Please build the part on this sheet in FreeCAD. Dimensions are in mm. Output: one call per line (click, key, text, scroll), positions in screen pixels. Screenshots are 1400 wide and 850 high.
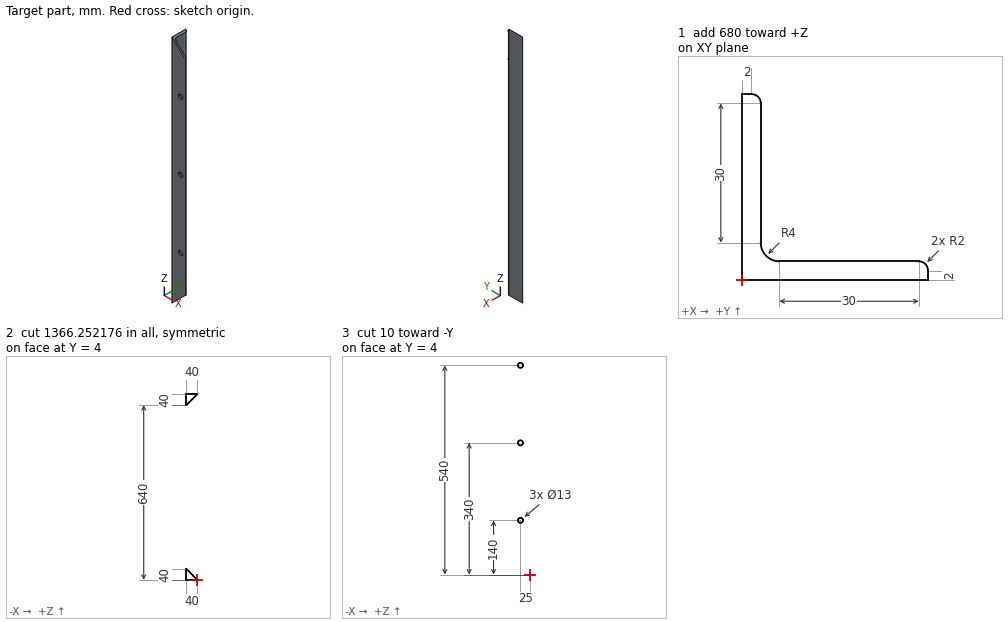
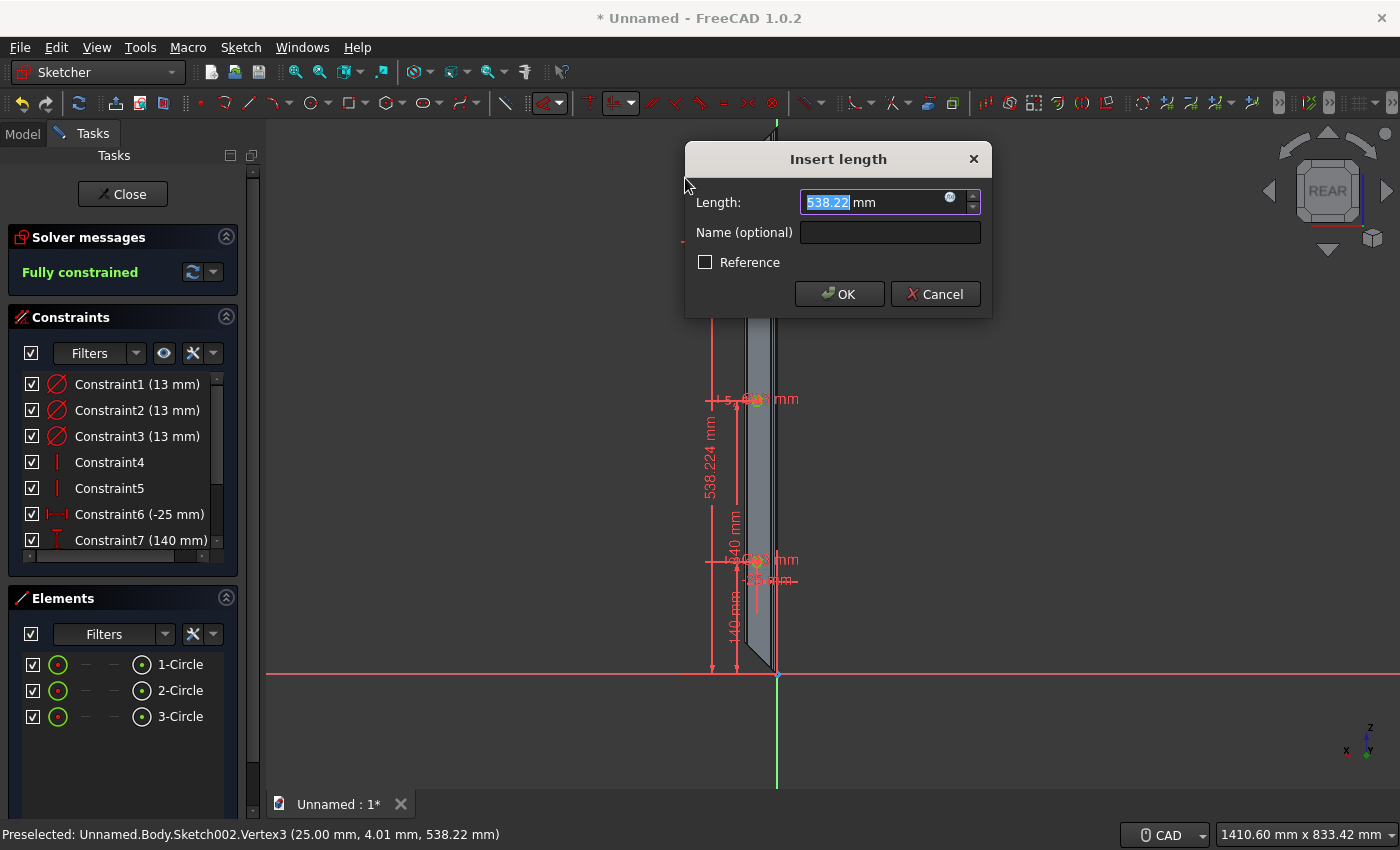
text(540)
key(Return)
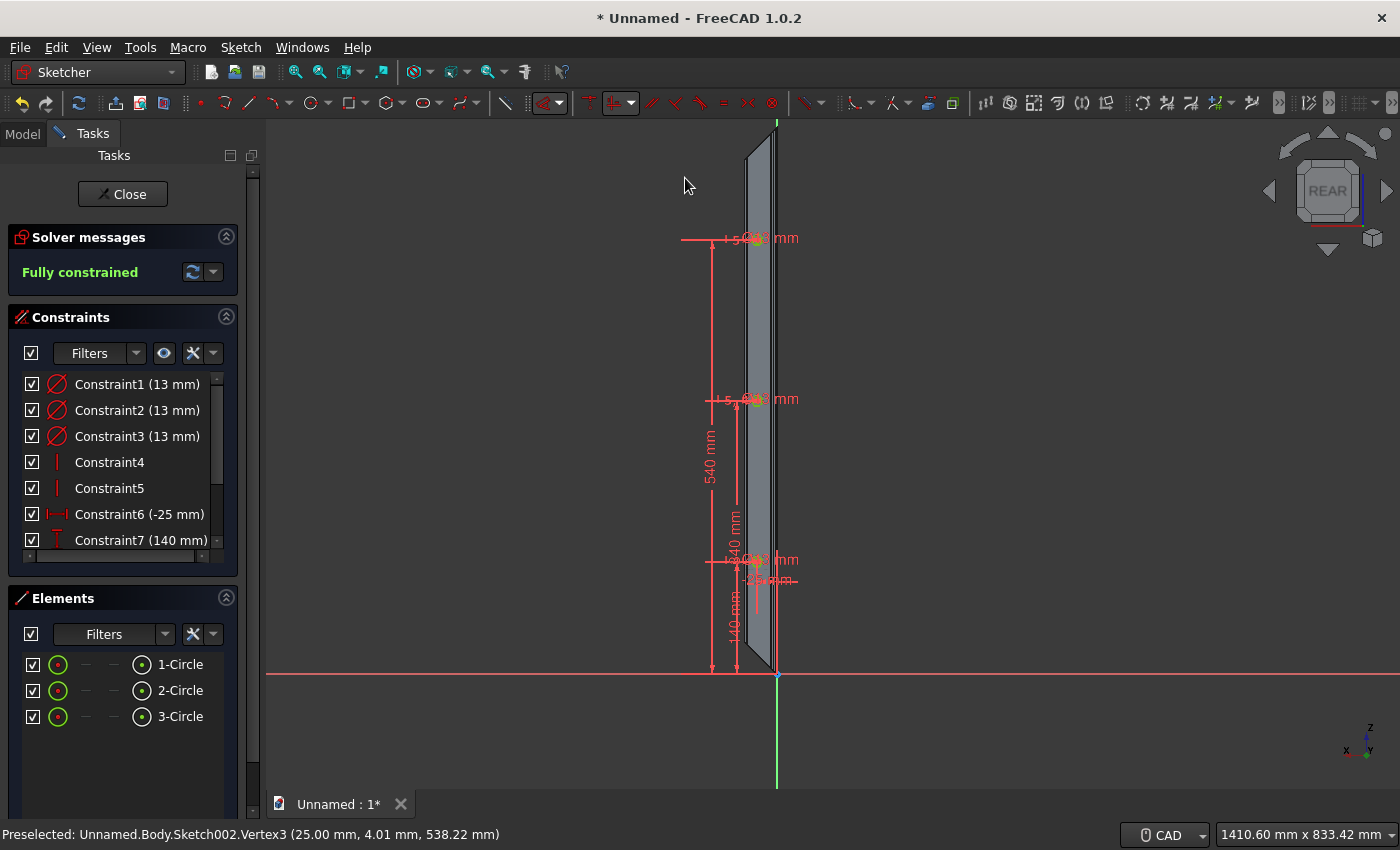
click(123, 194)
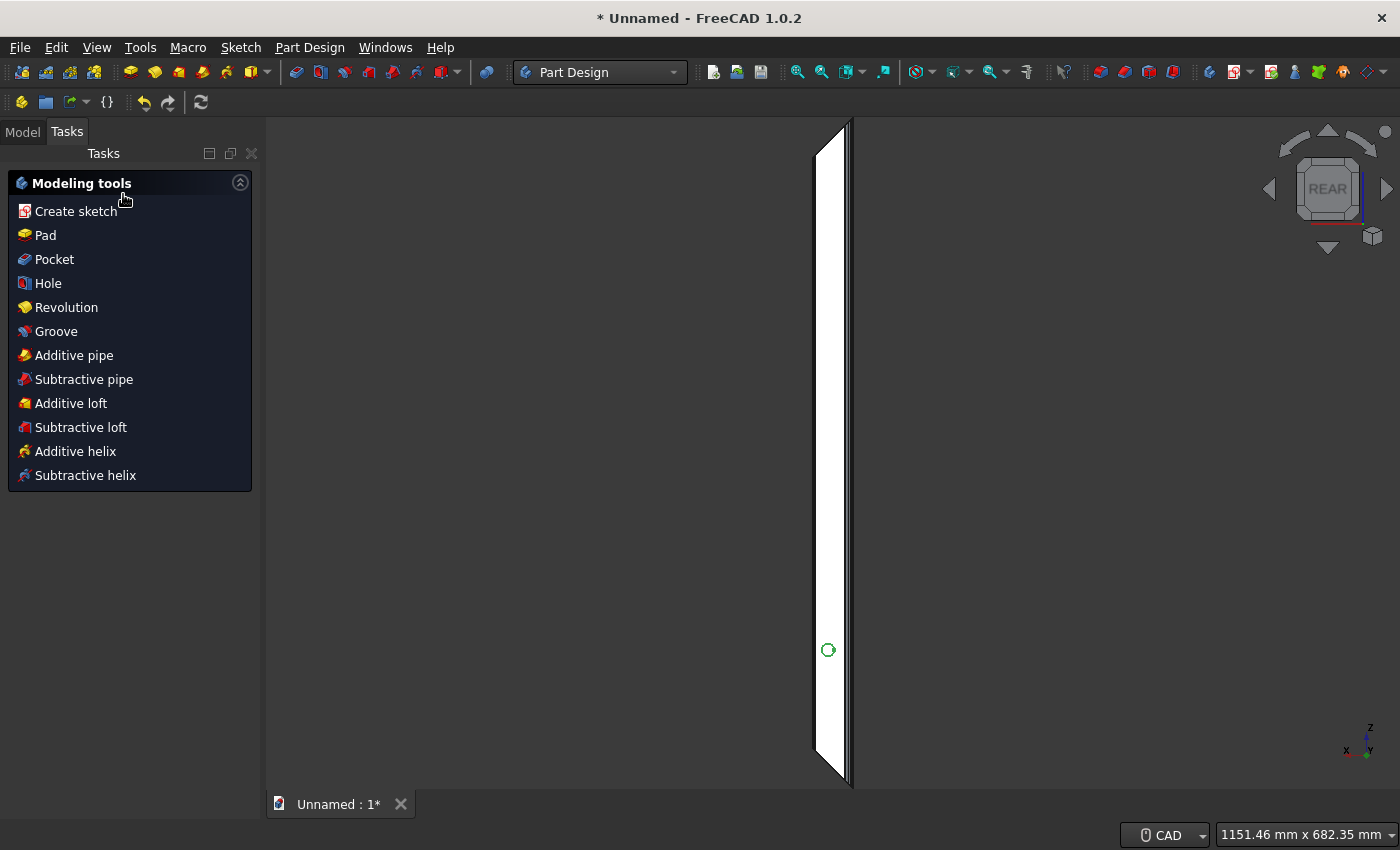
click(298, 72)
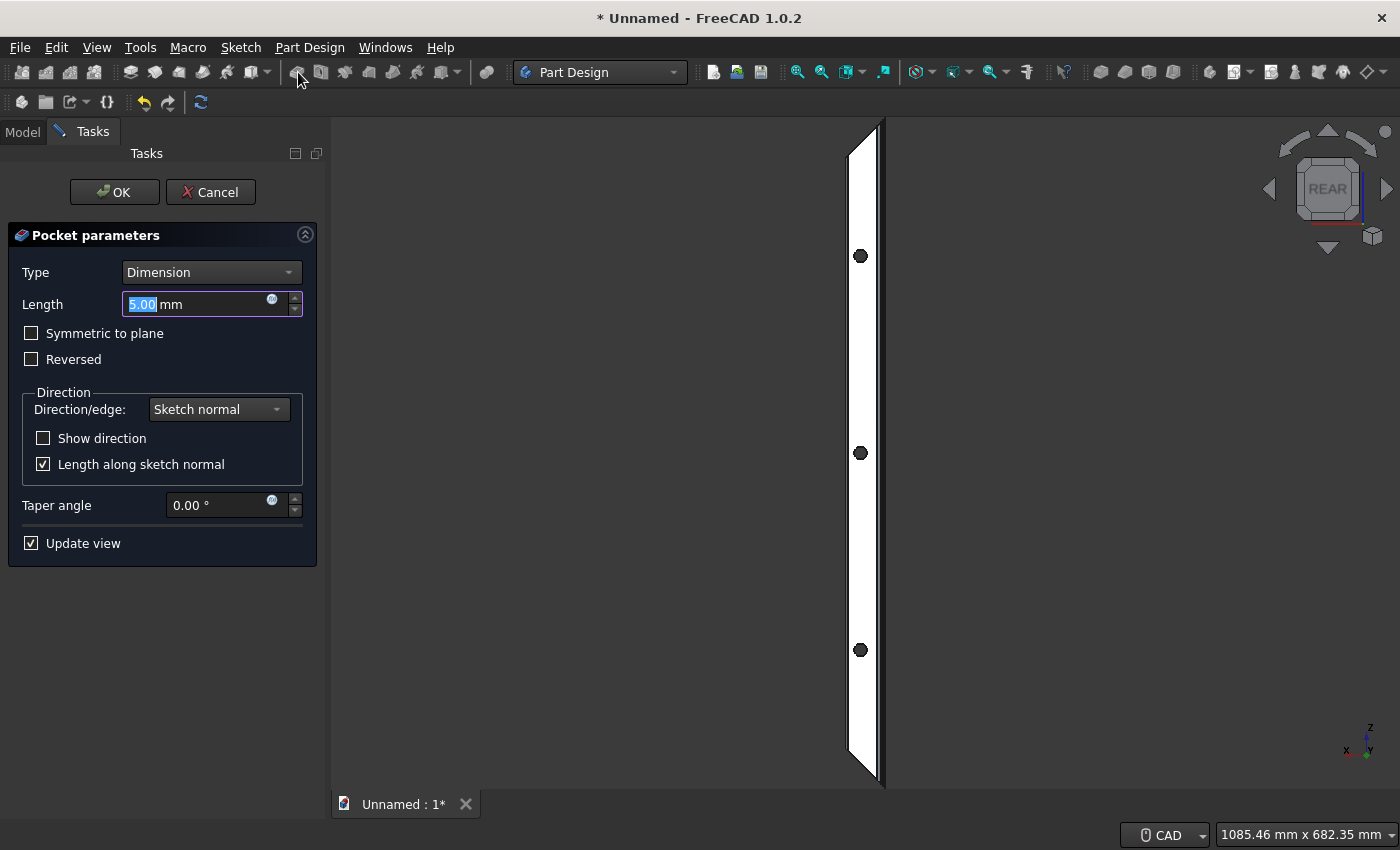
text(10)
key(Tab)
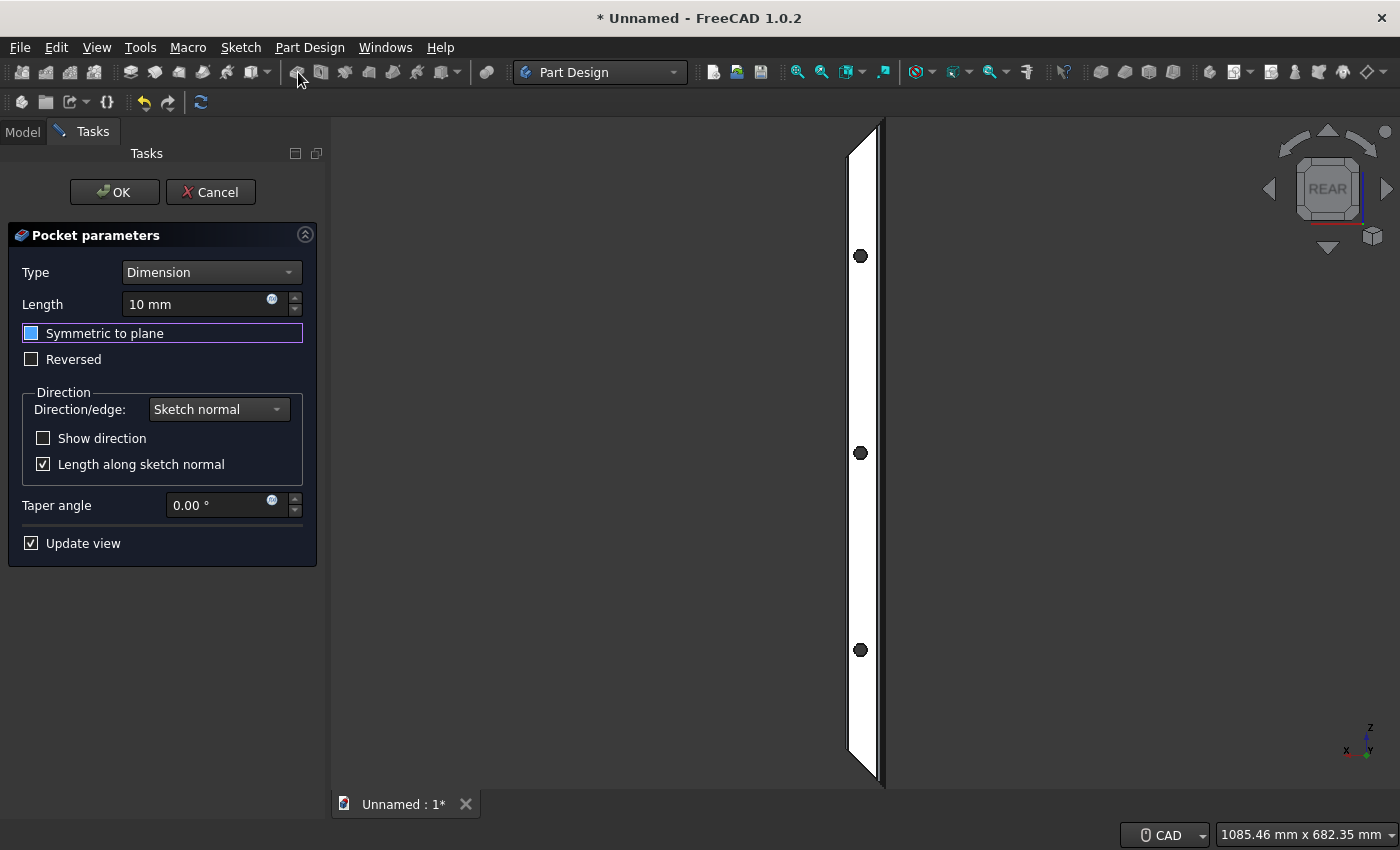
click(115, 192)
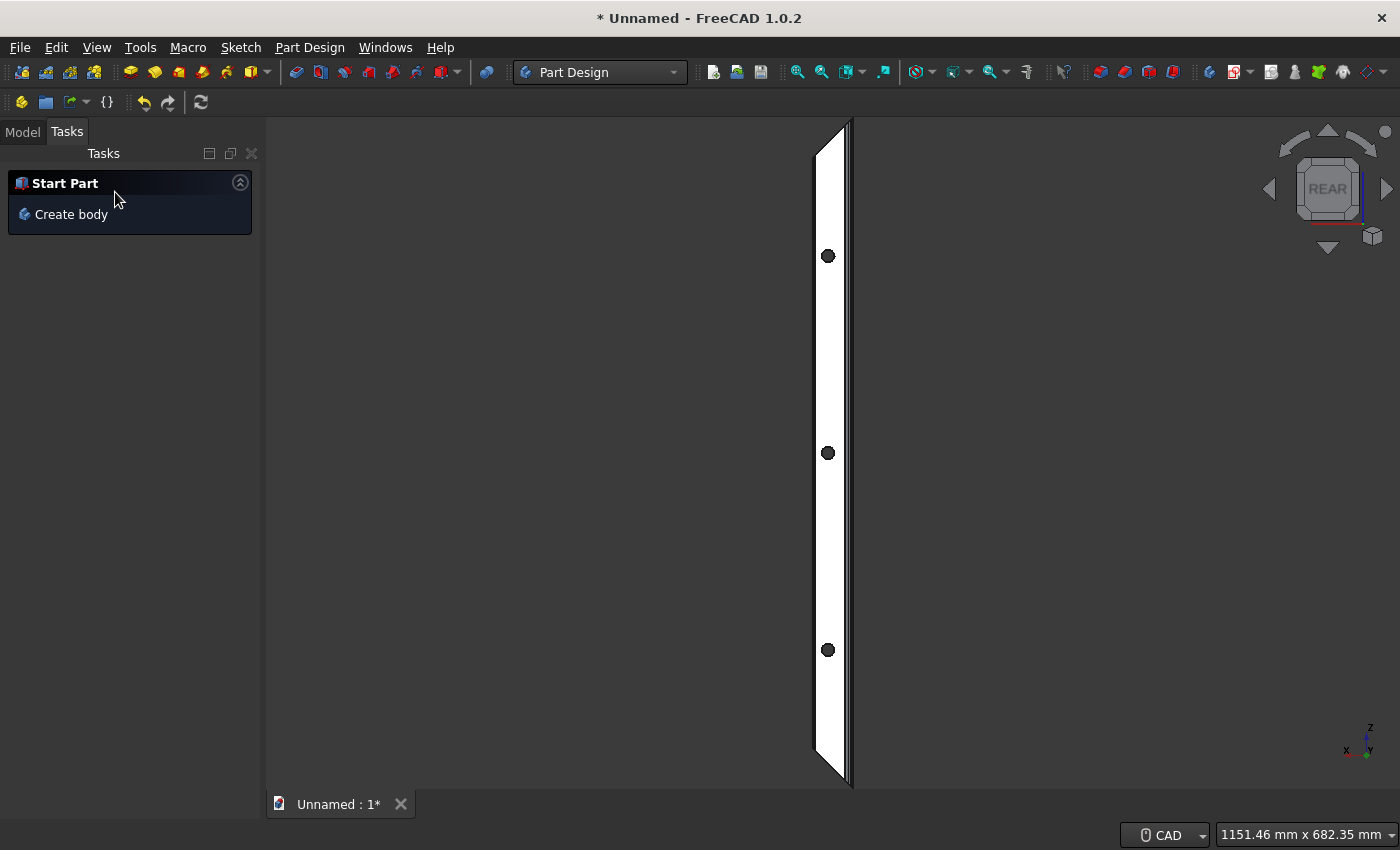
key(0)